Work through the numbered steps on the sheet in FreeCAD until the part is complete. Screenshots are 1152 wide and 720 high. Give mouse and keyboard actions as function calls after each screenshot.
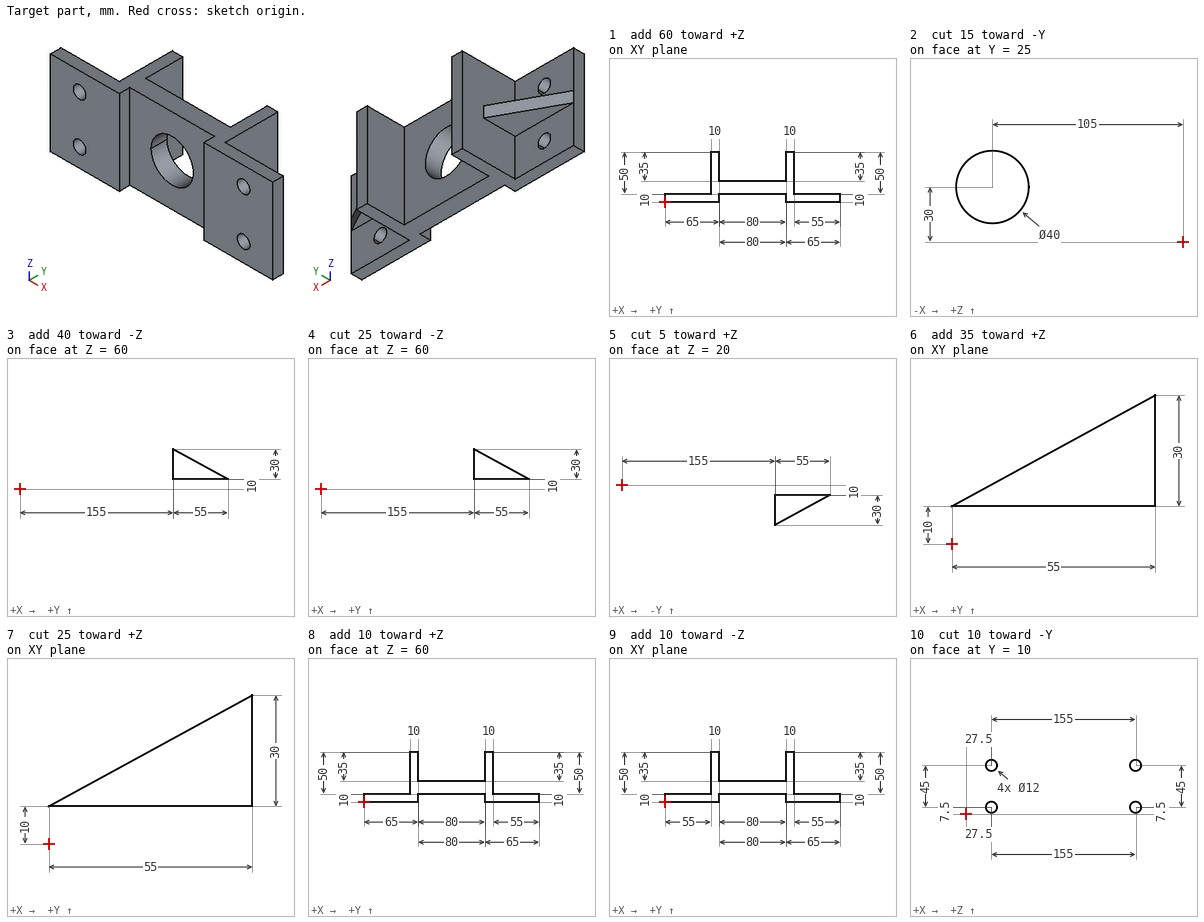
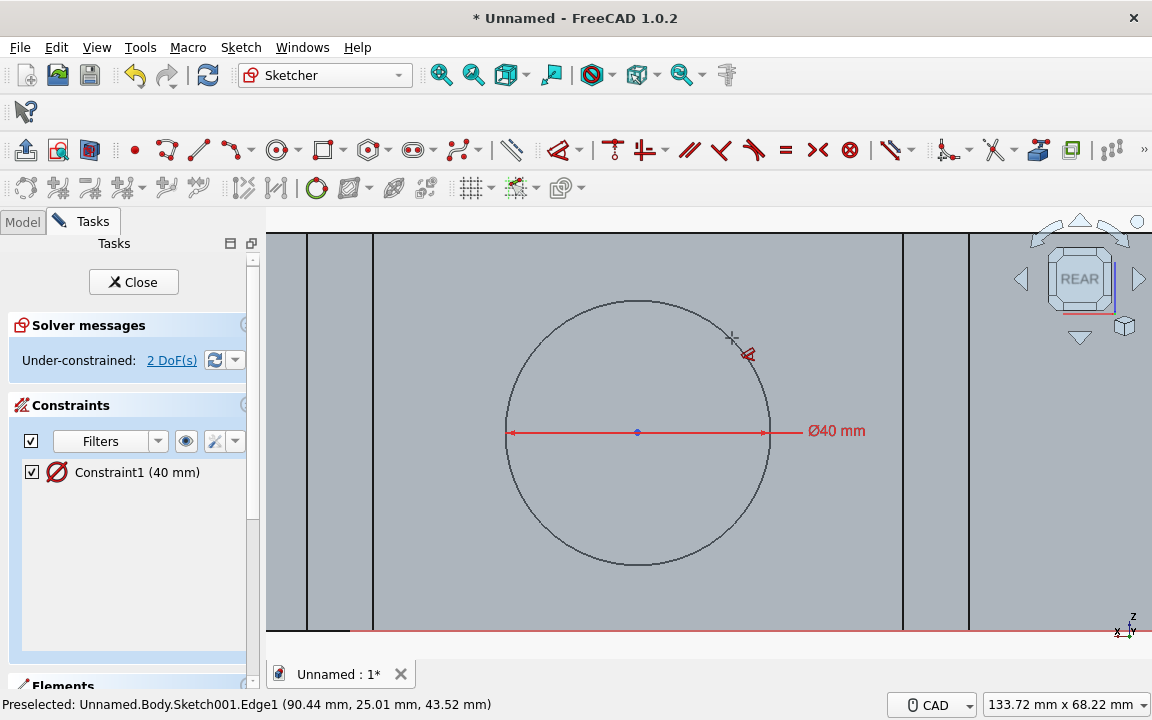
click(638, 433)
click(604, 532)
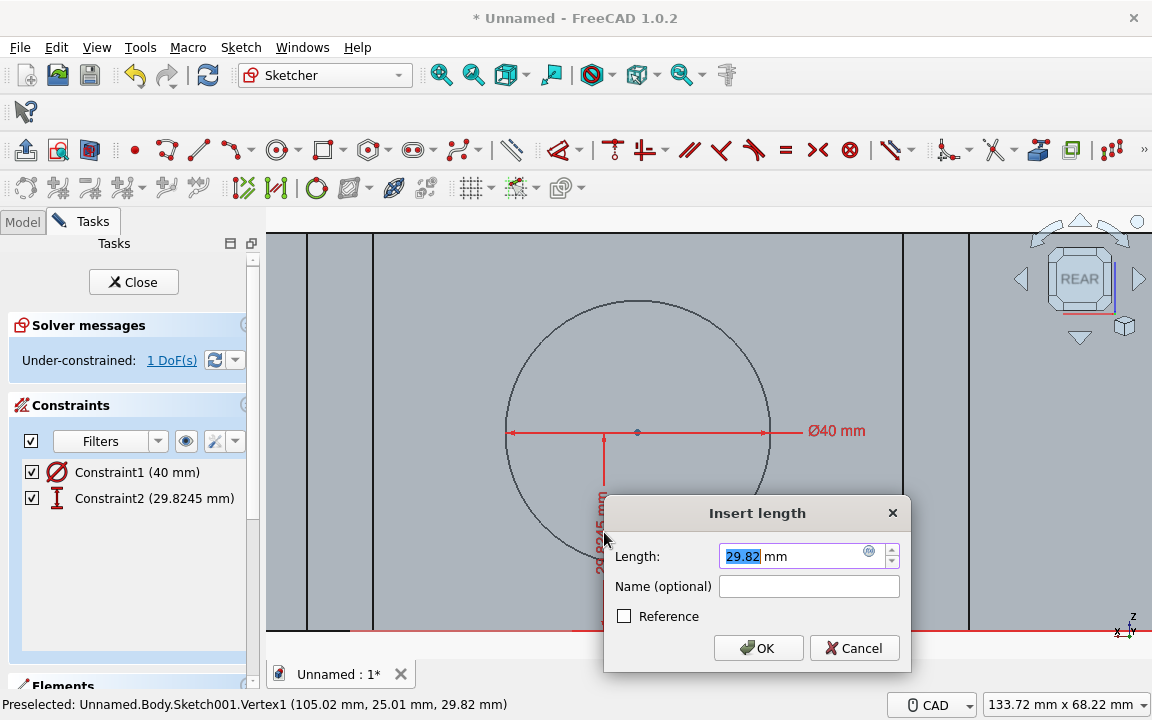
text(30)
key(Return)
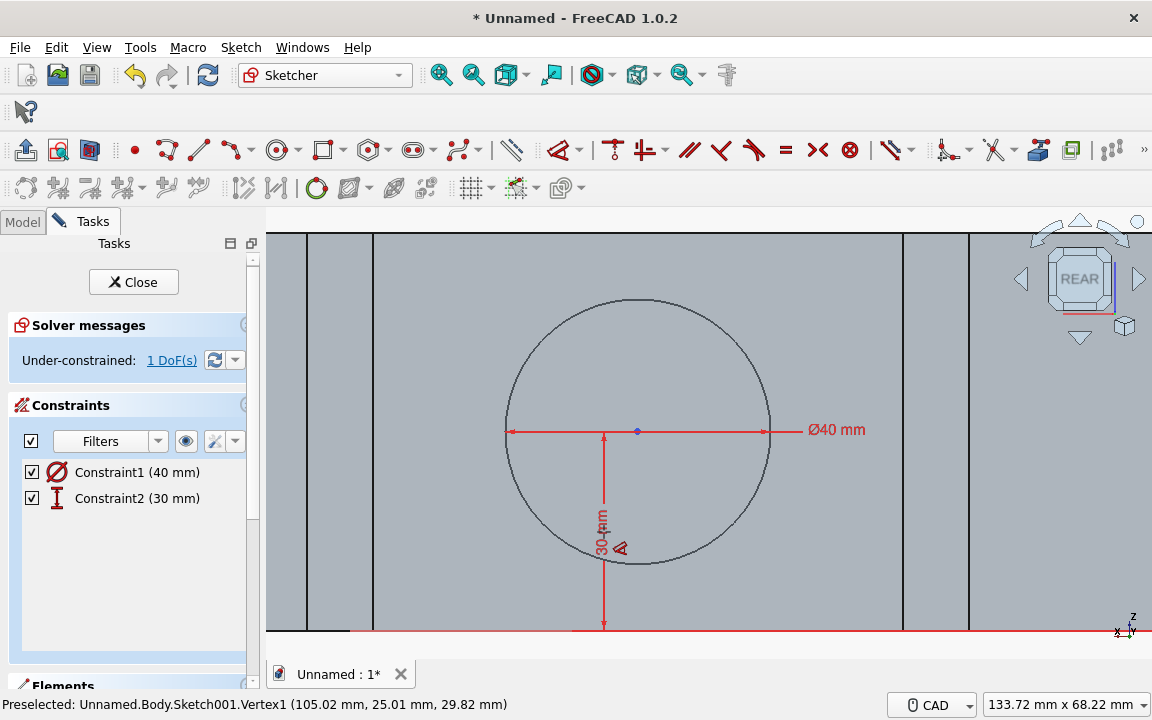
click(638, 432)
click(813, 398)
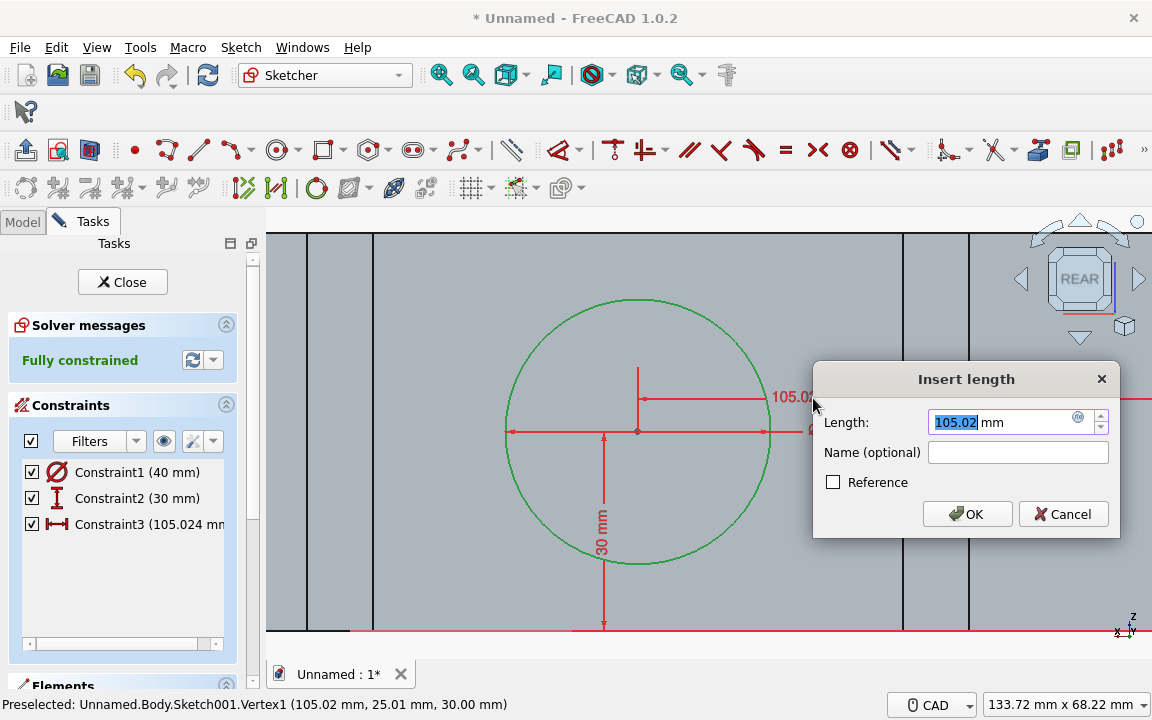
text(105)
key(Return)
key(Escape)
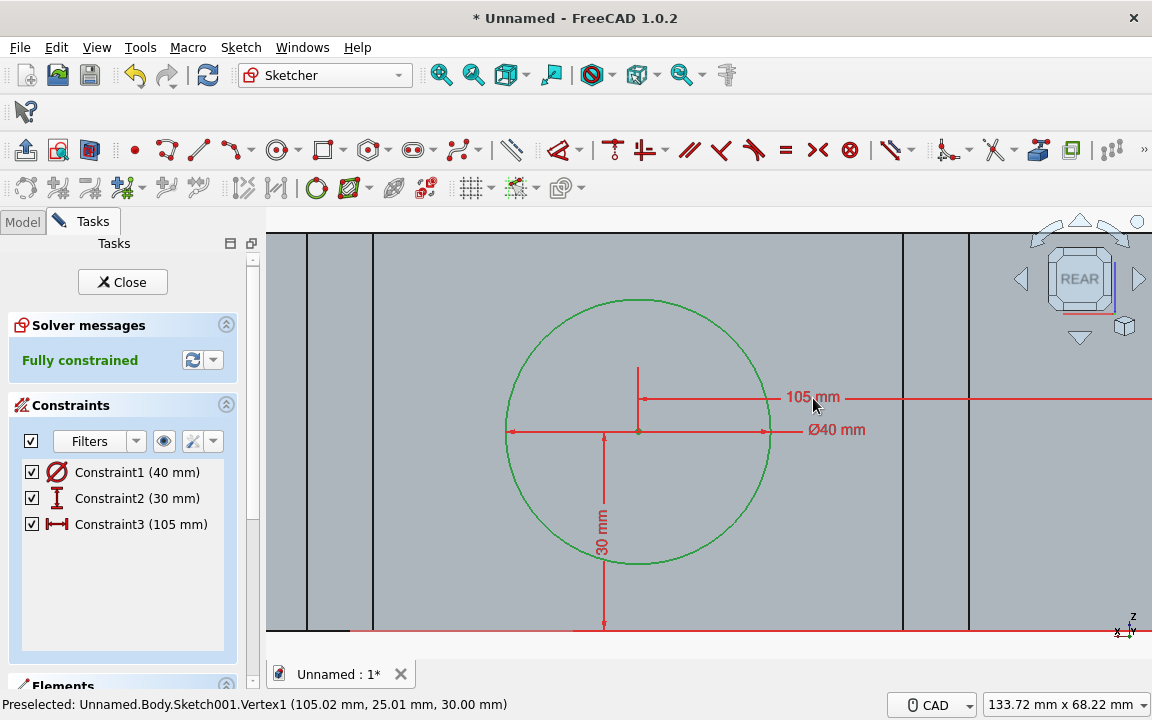
click(123, 282)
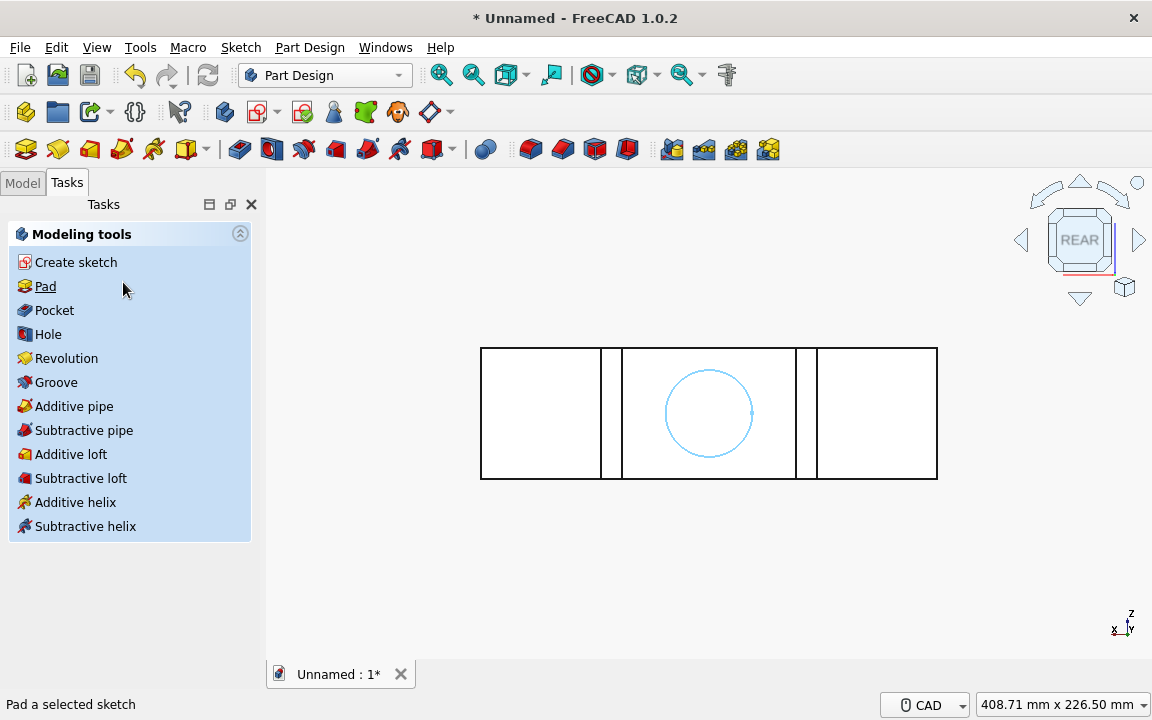
click(240, 150)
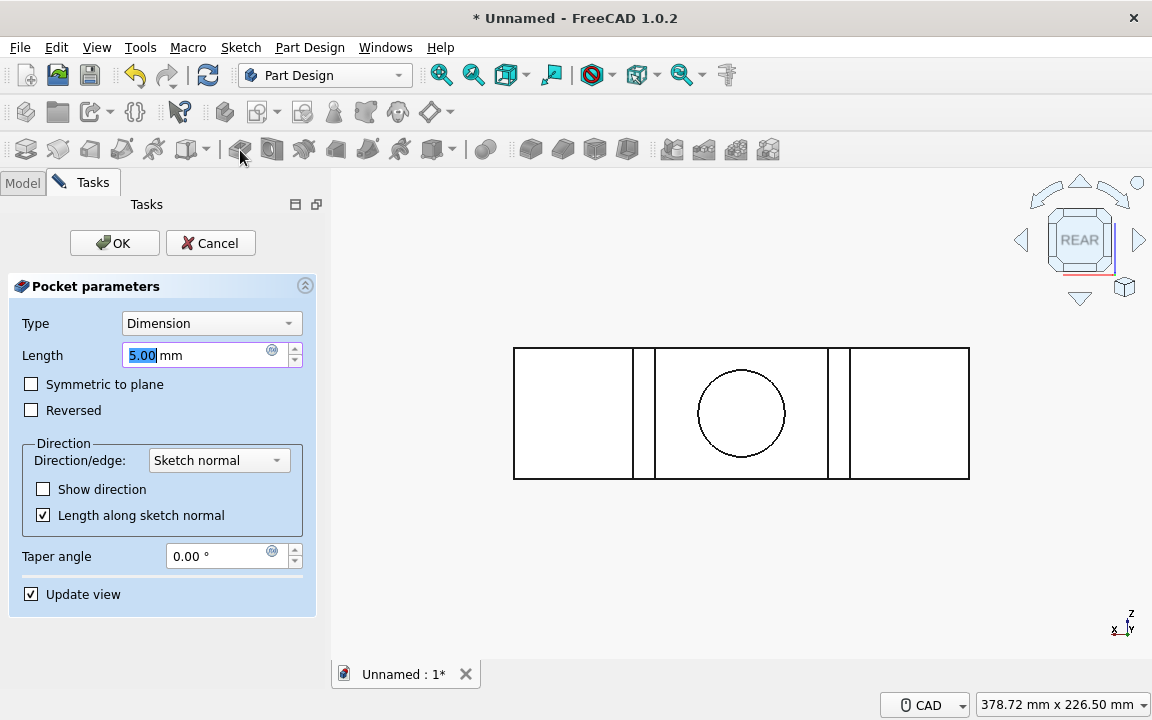
text(15)
key(Tab)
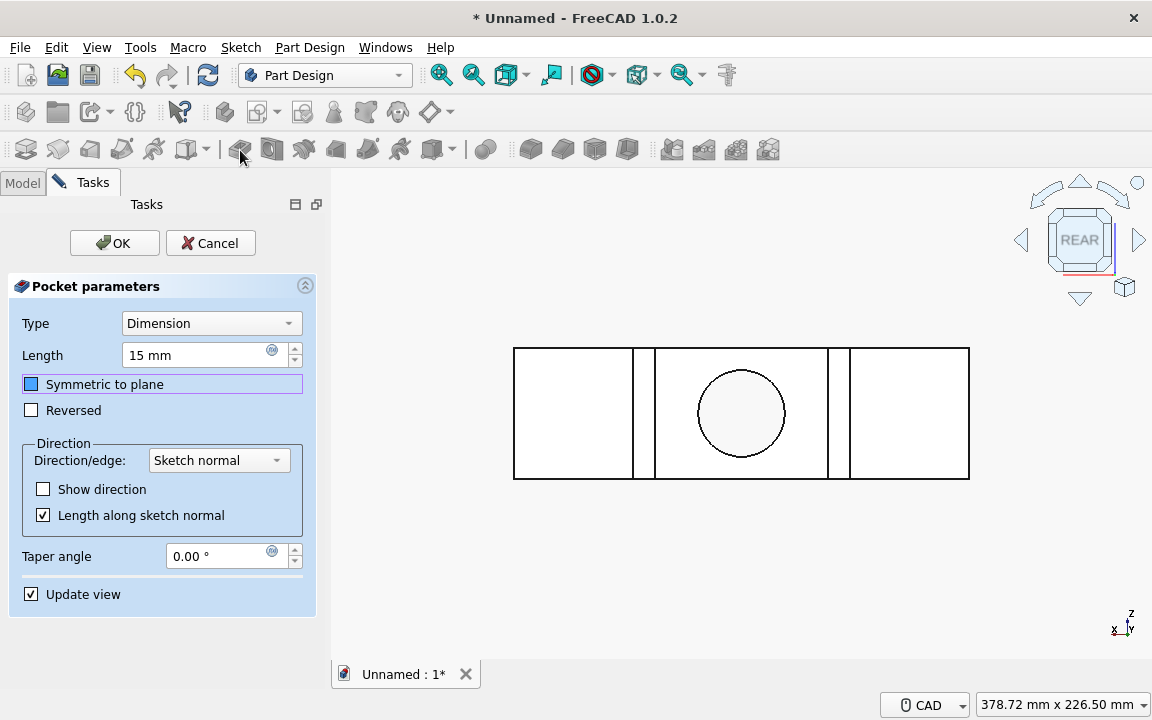
click(115, 243)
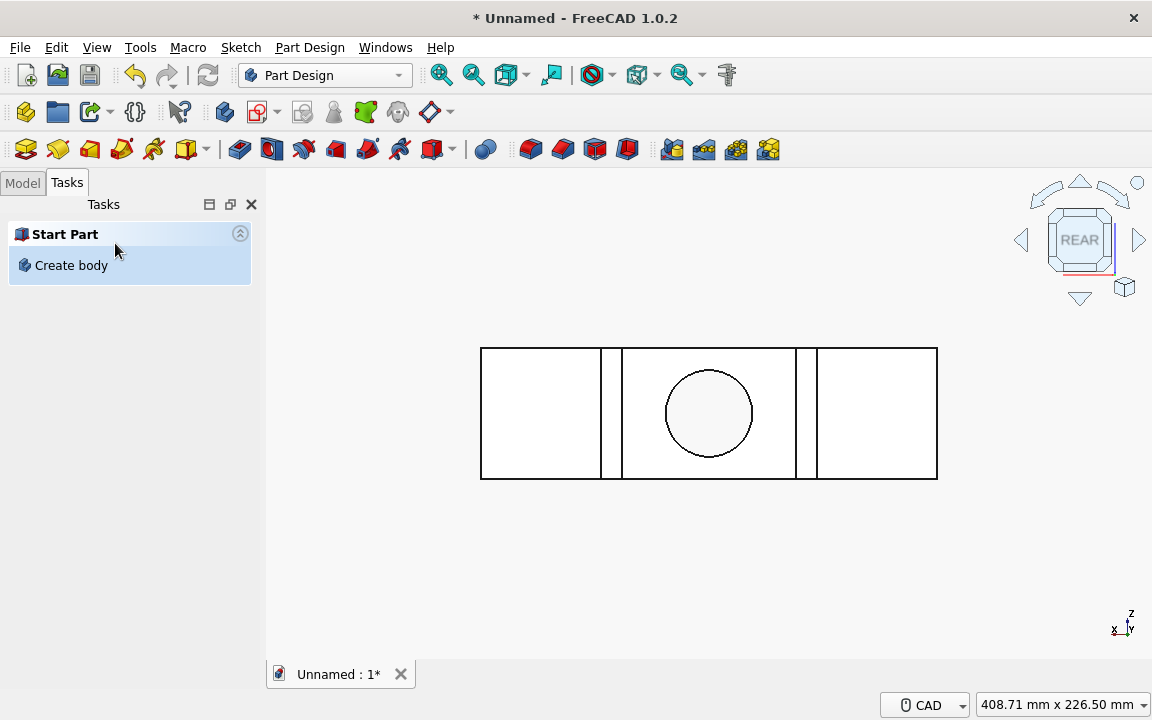
key(0)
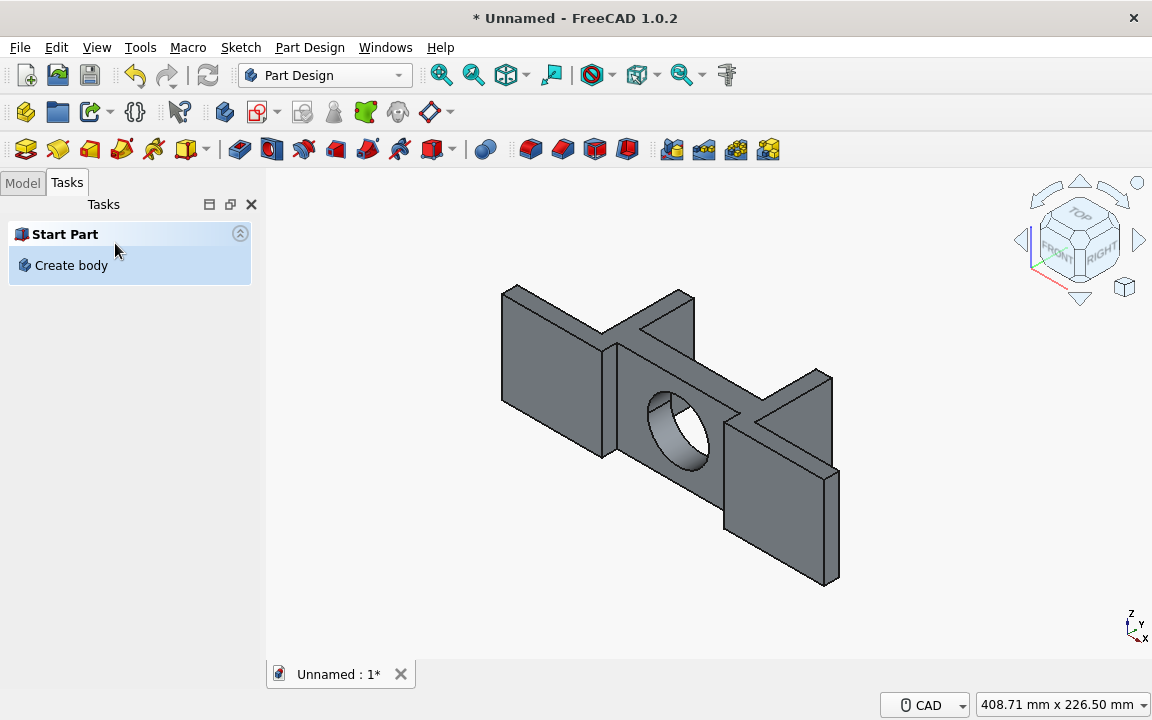
click(742, 394)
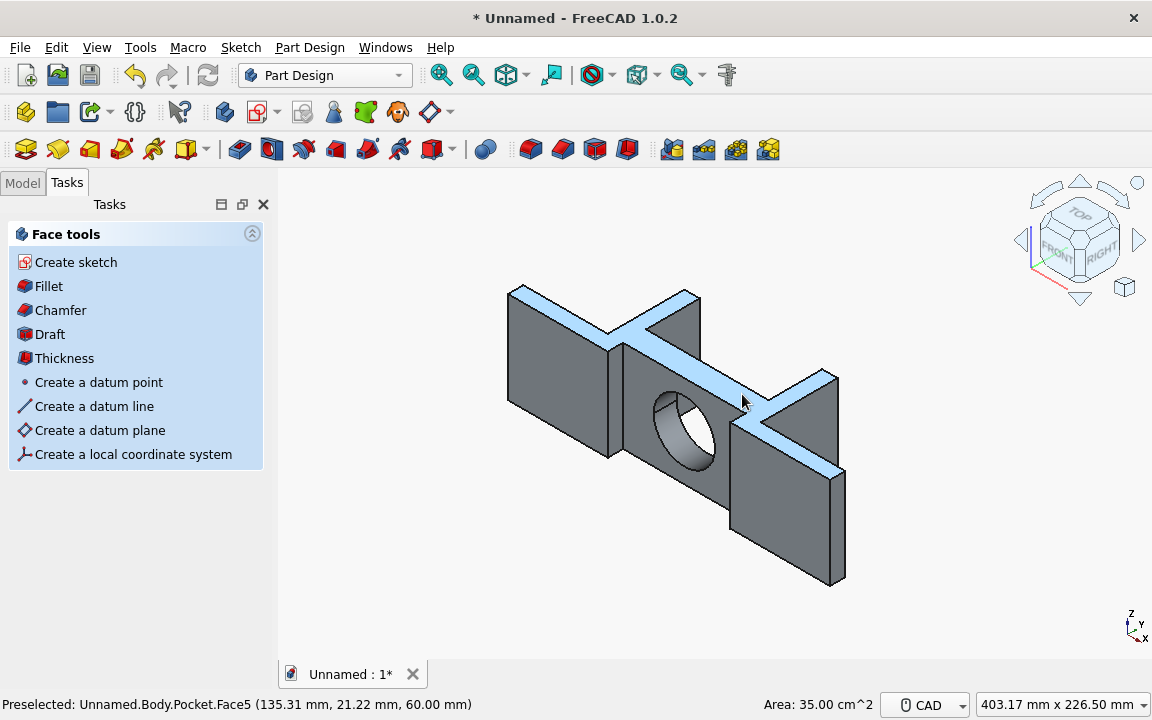
click(258, 112)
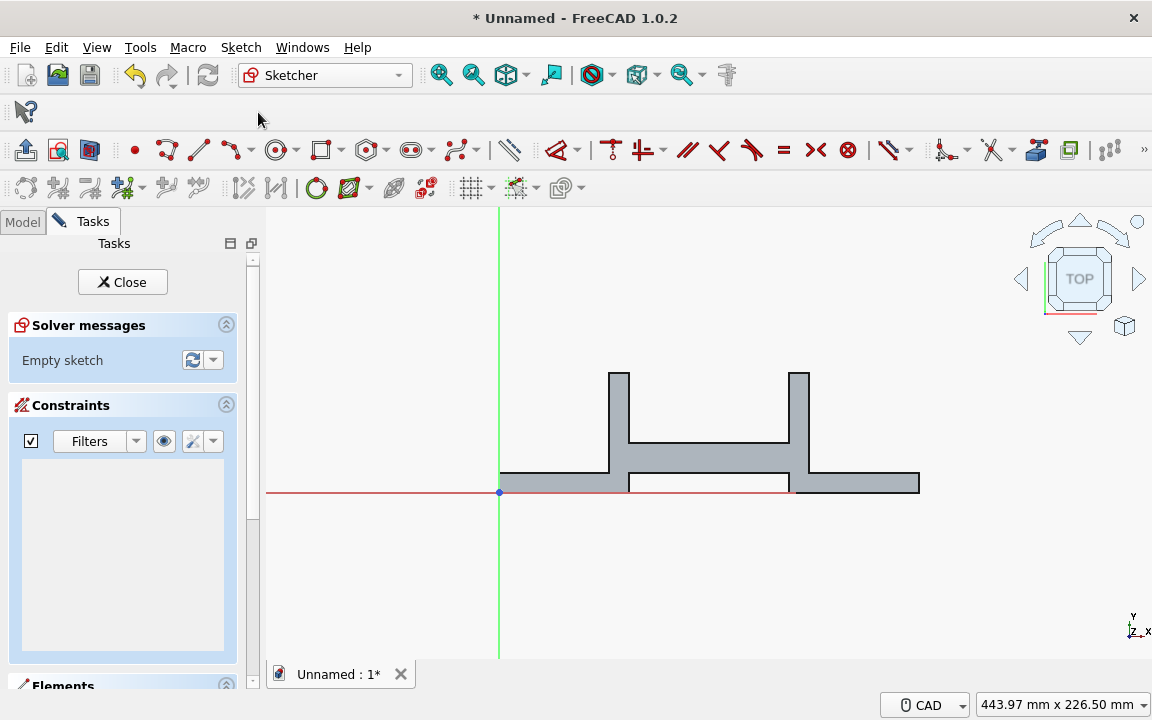
scroll(937, 446, up, 7)